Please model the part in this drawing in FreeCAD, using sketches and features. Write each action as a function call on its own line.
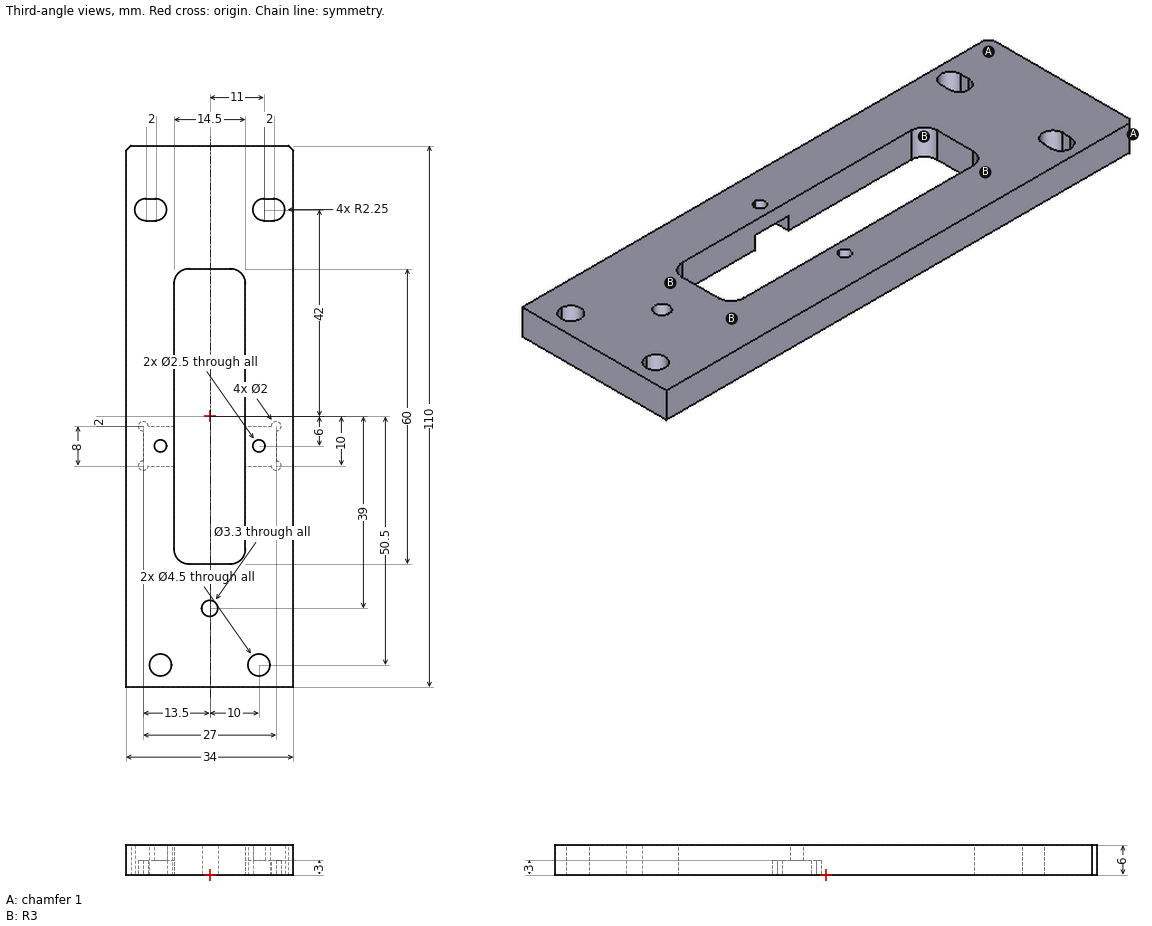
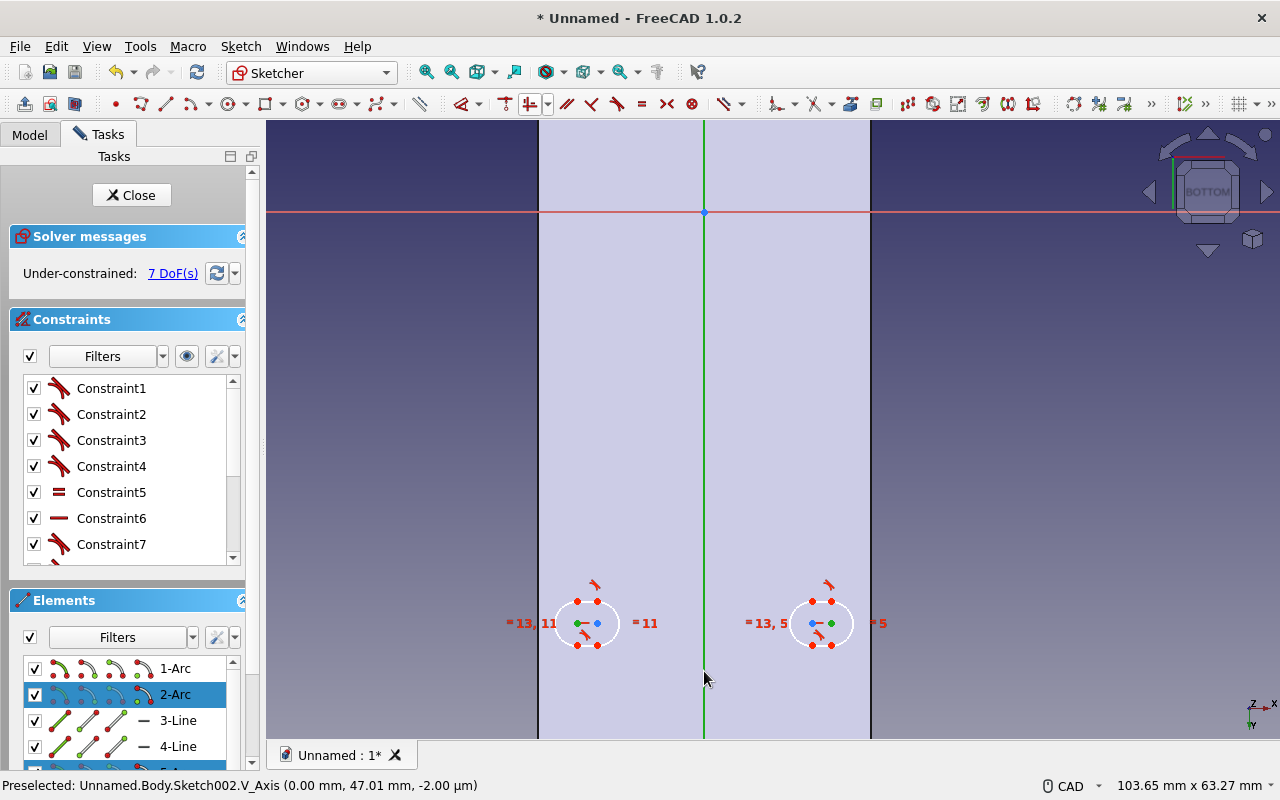
click(667, 104)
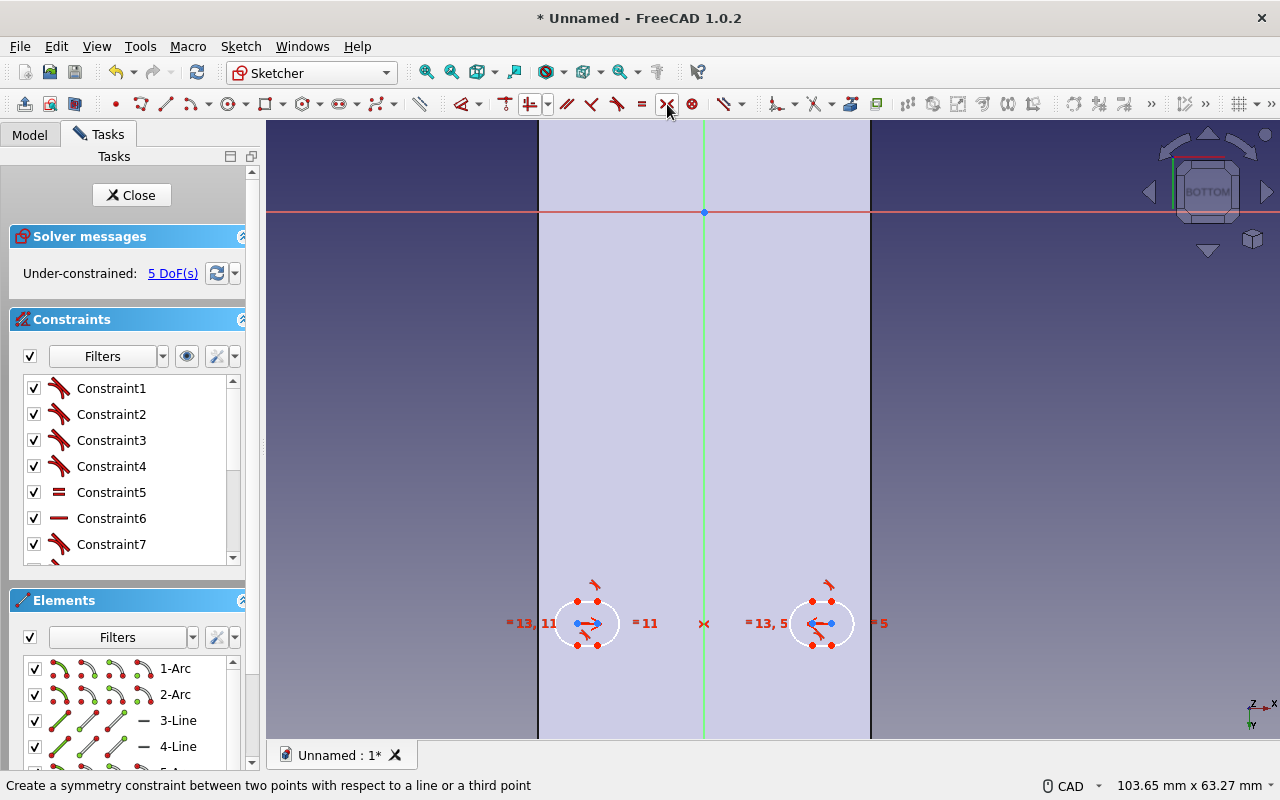
scroll(794, 611, up, 3)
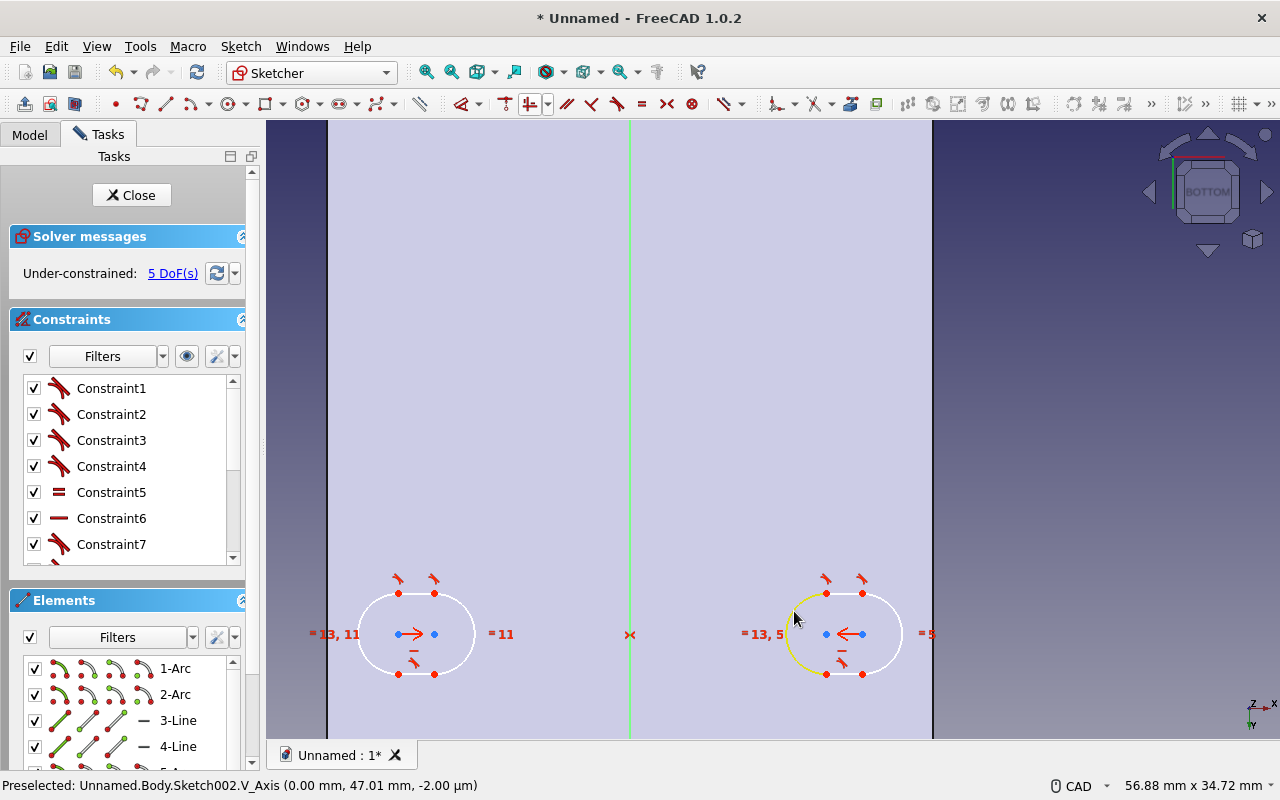
click(794, 610)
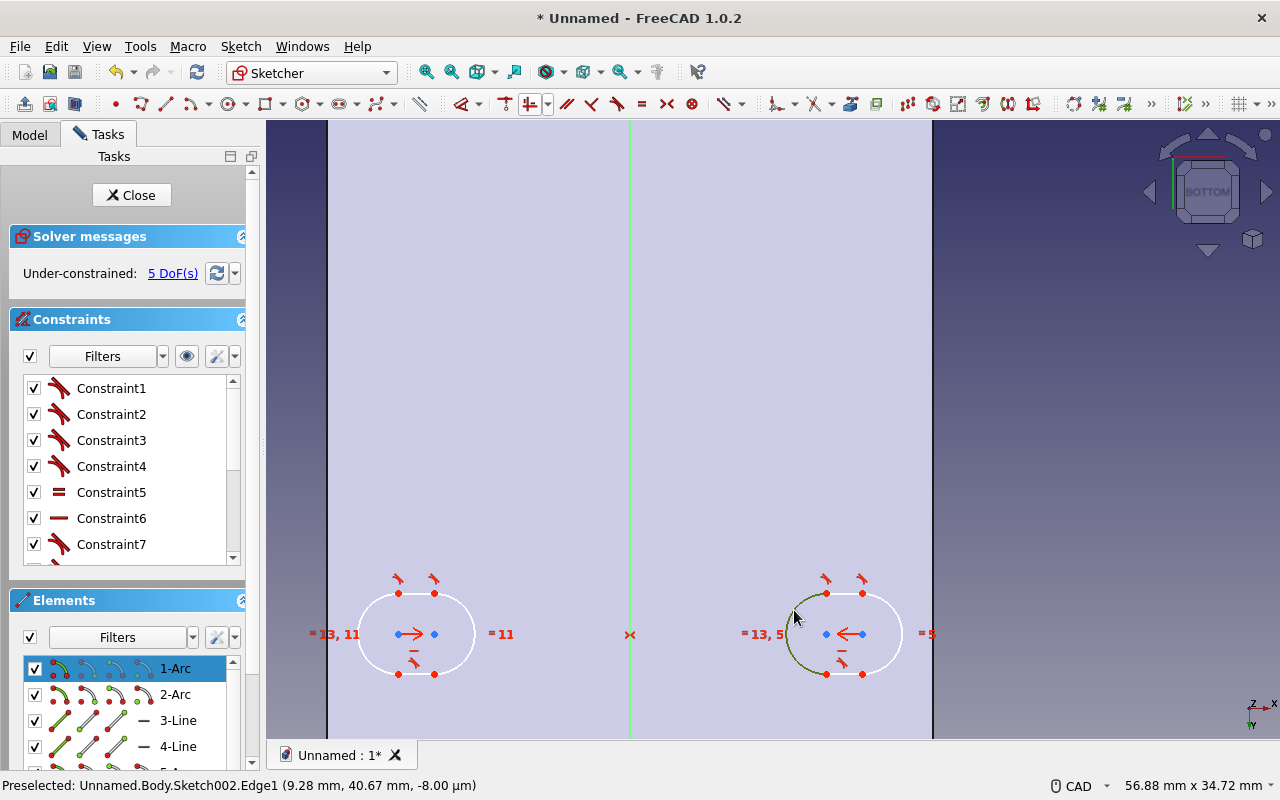
key(k)
key(r)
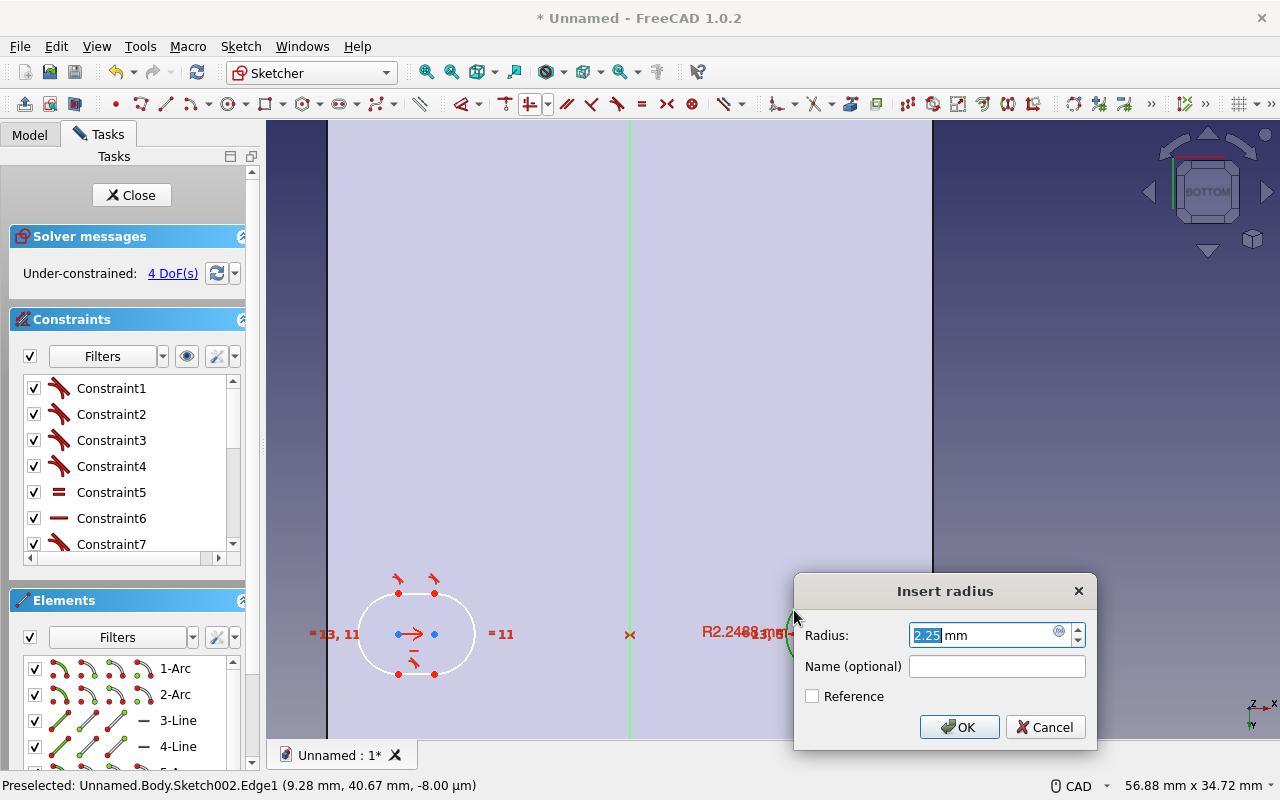
text(2.25)
key(Return)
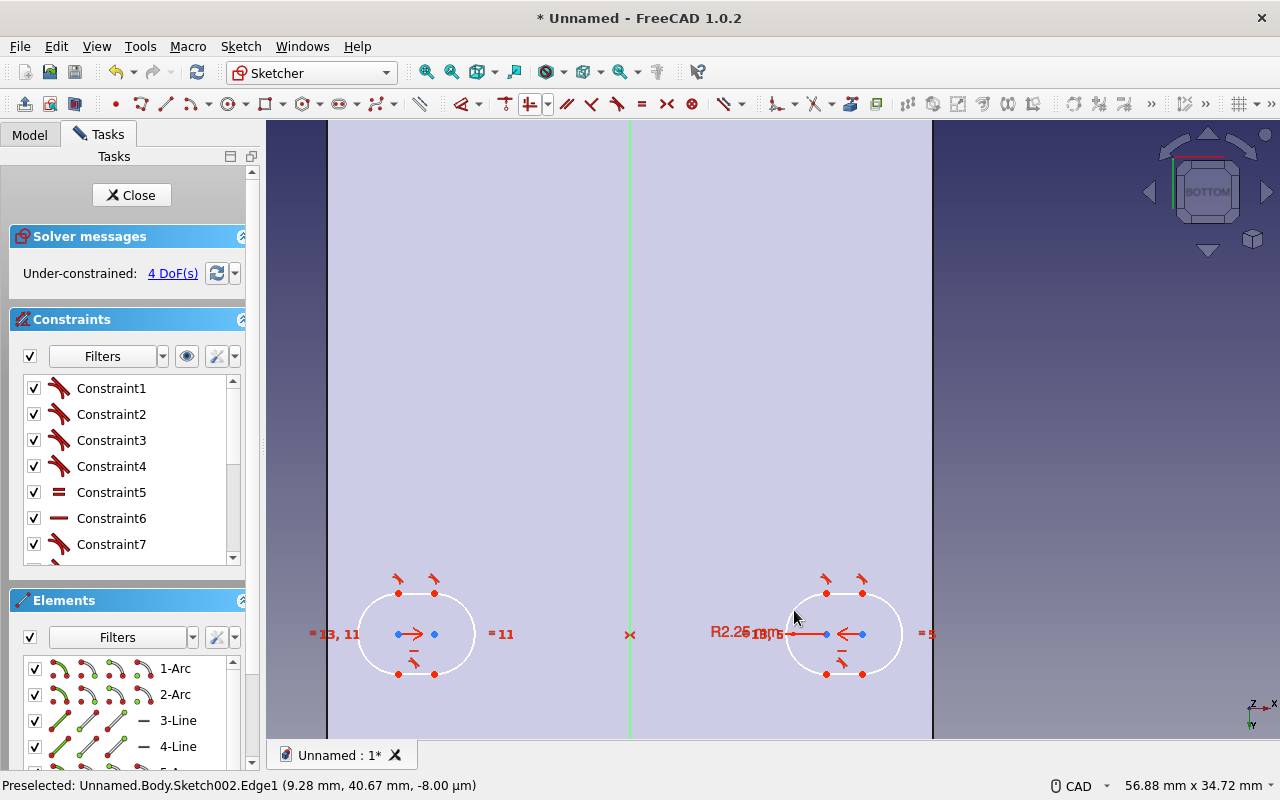
scroll(837, 594, up, 2)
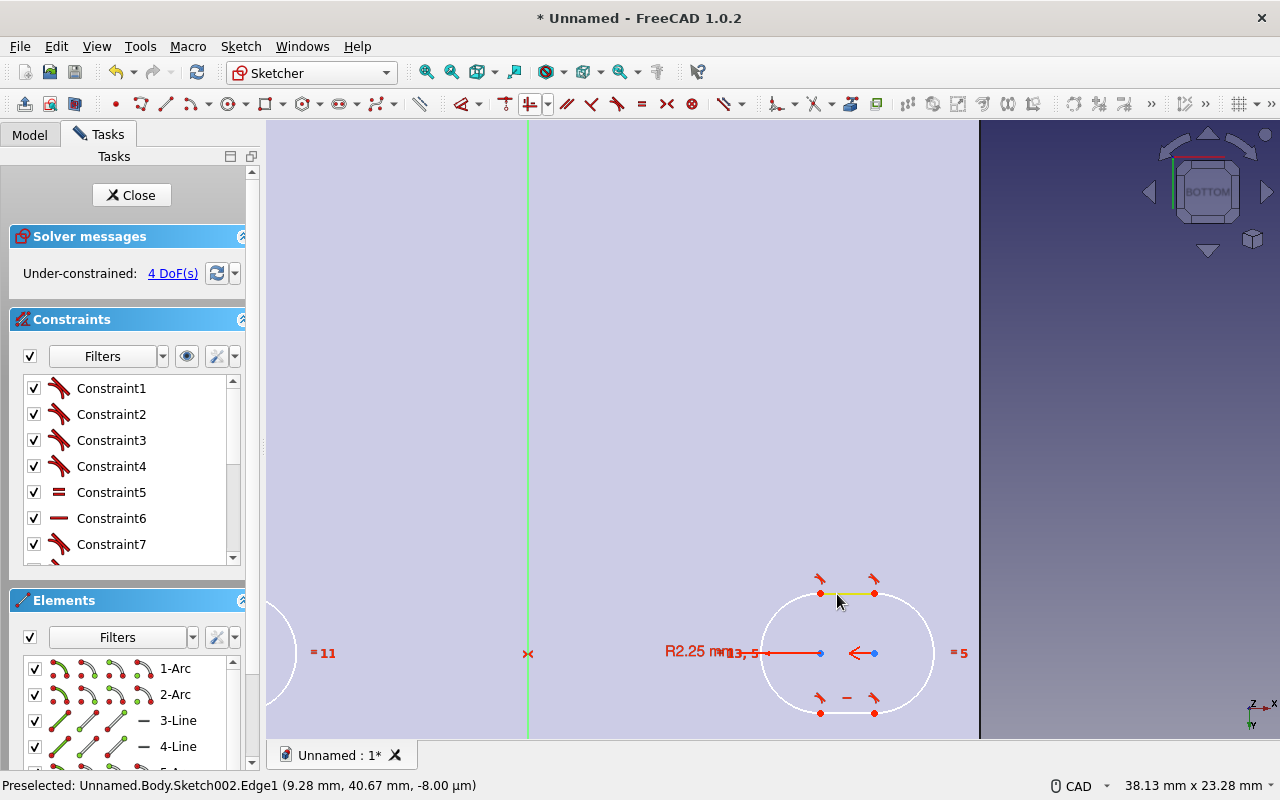
click(837, 594)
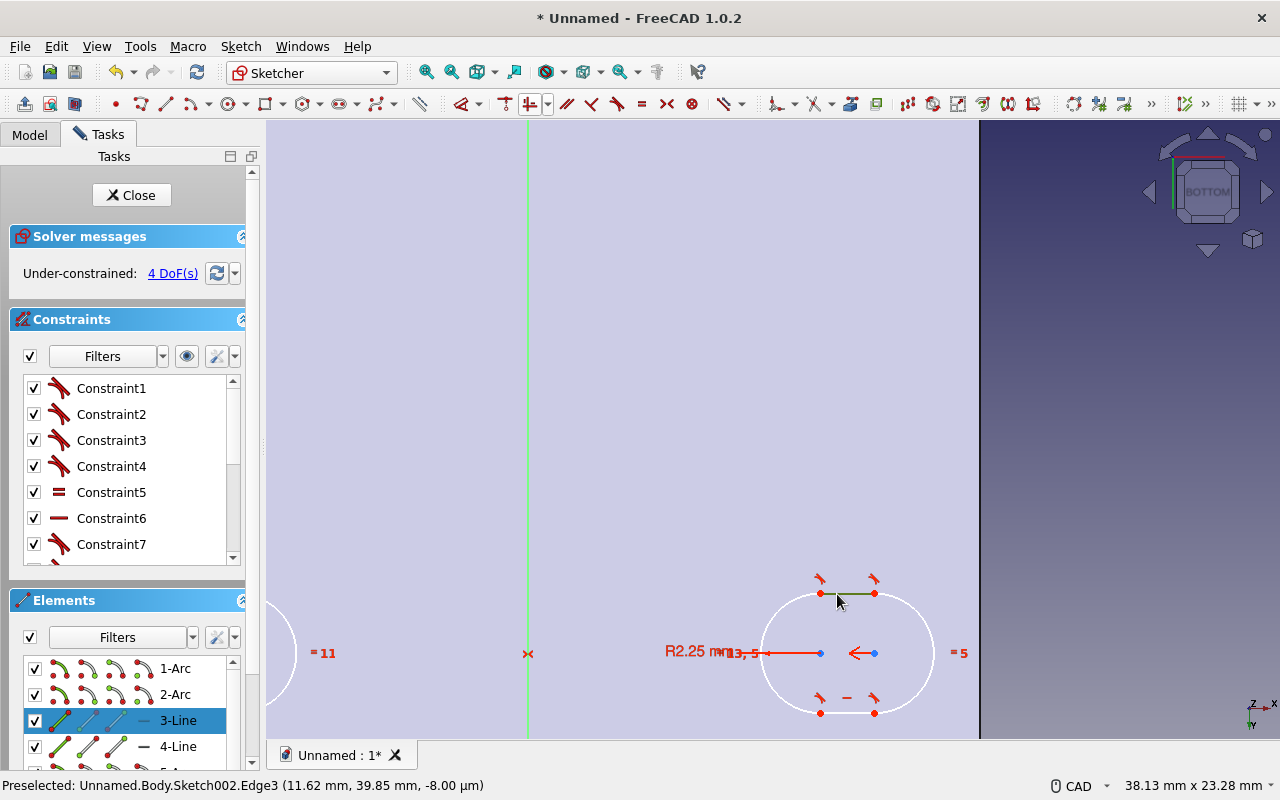
click(478, 104)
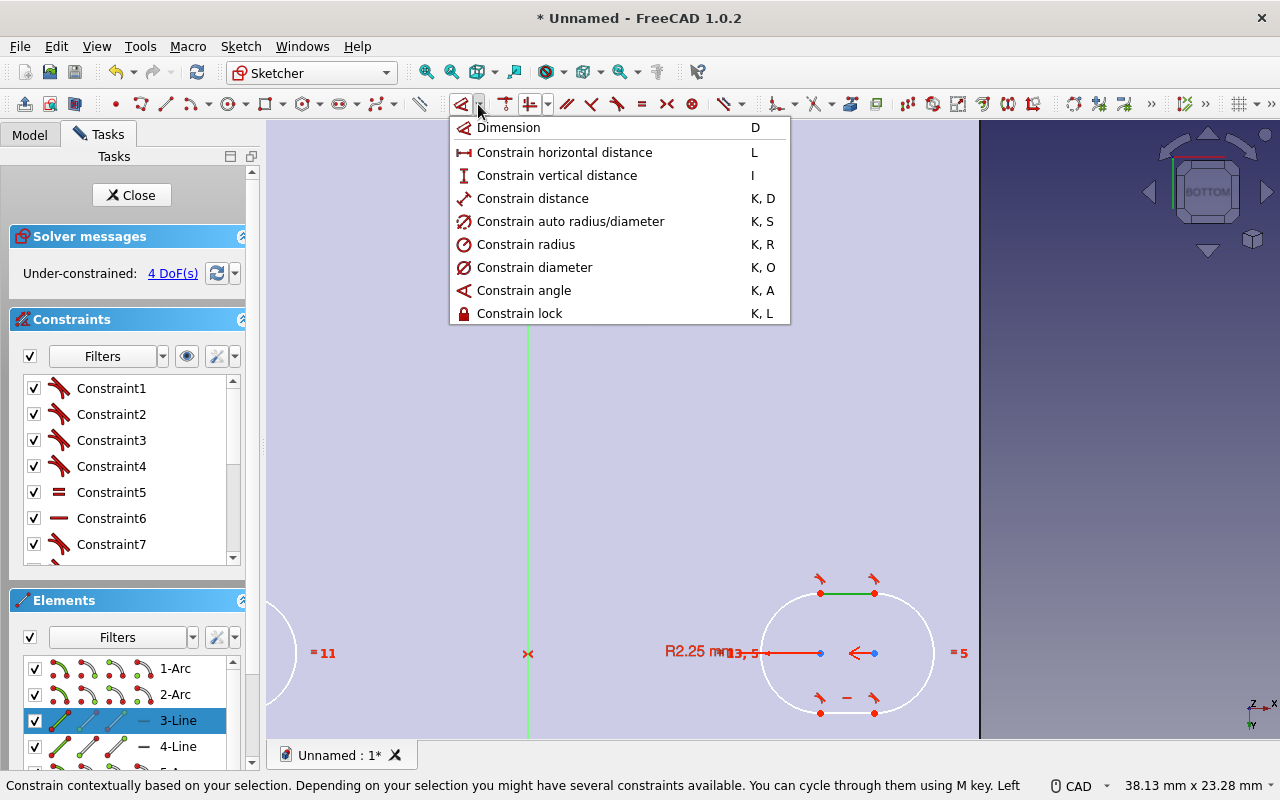
click(620, 152)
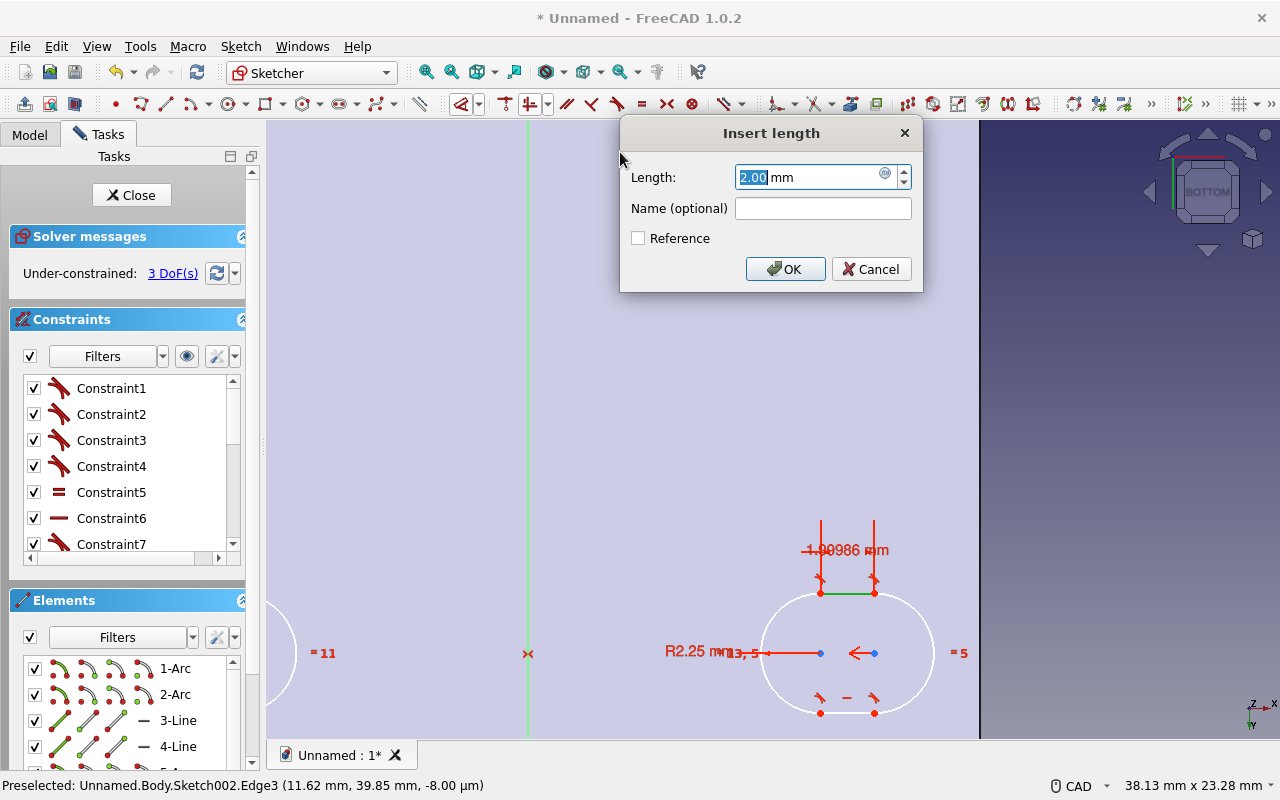
text(2)
key(Return)